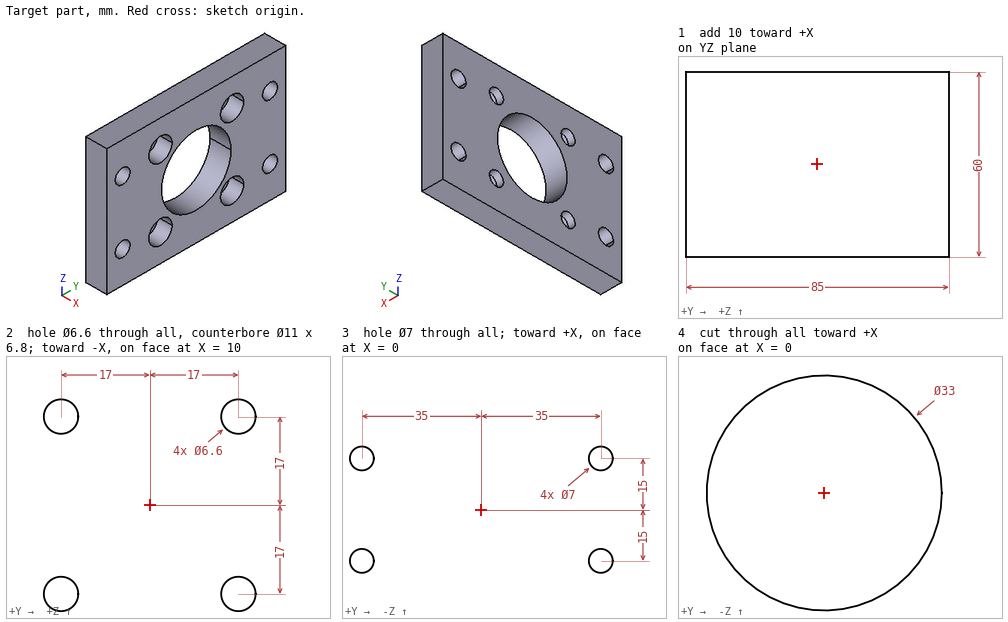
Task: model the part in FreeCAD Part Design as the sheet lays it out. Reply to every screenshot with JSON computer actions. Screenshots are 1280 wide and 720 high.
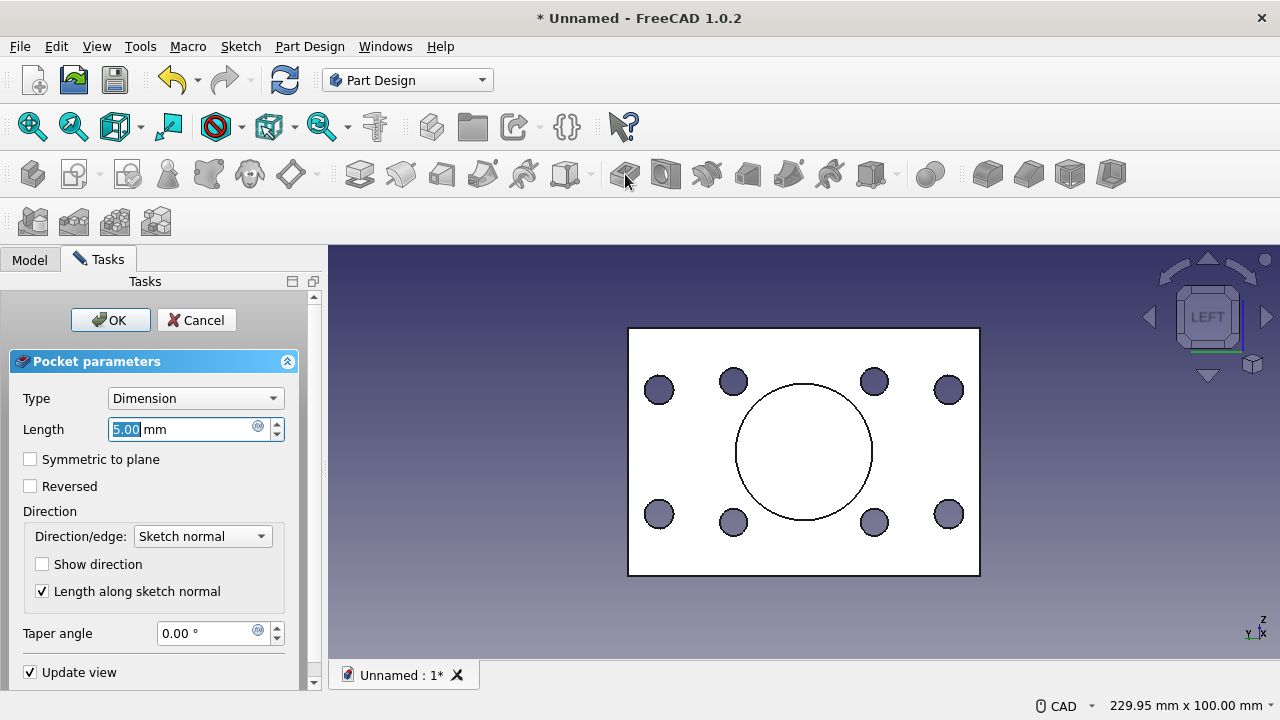
{"action": "left_click", "coordinate": [196, 398]}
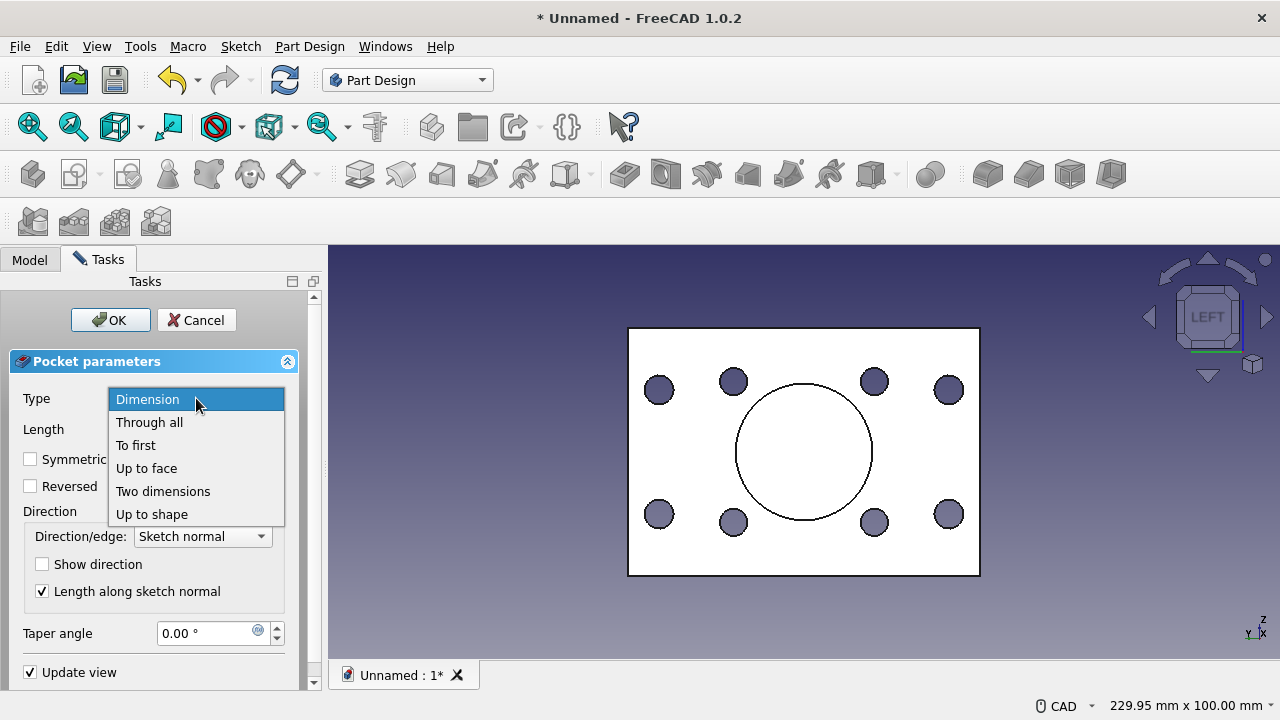
{"action": "left_click", "coordinate": [194, 422]}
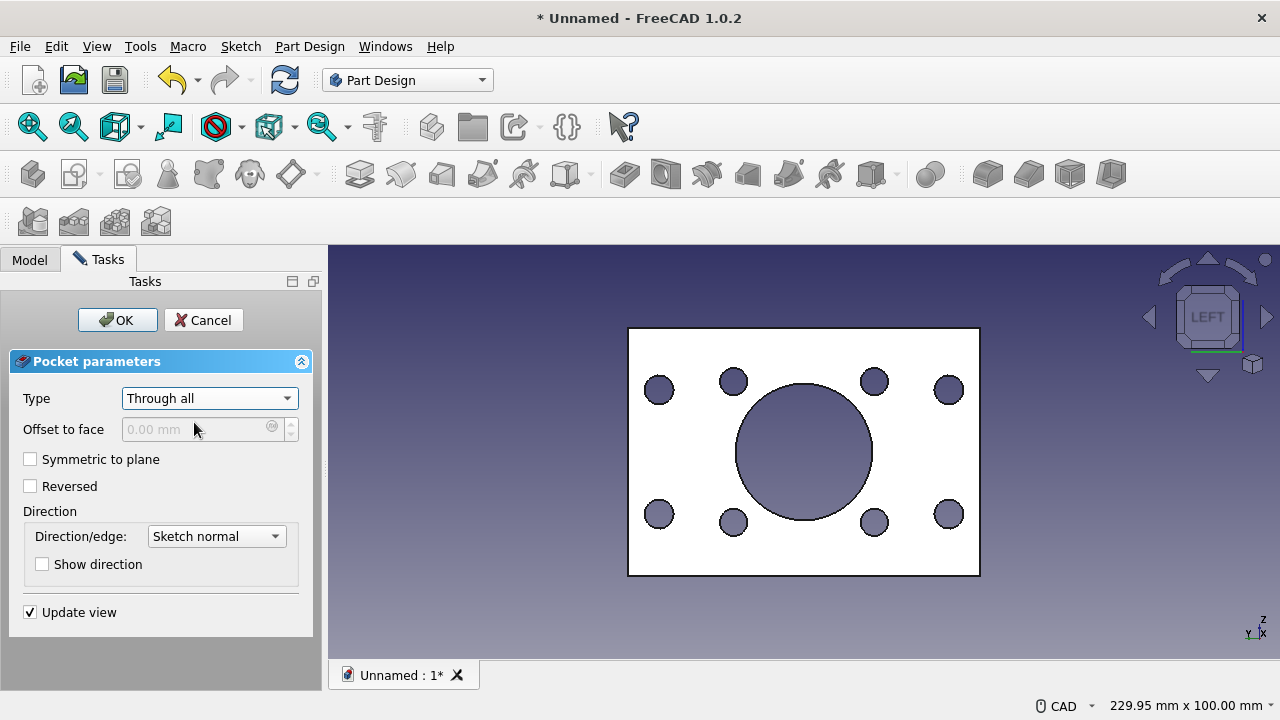
{"action": "left_click", "coordinate": [118, 320]}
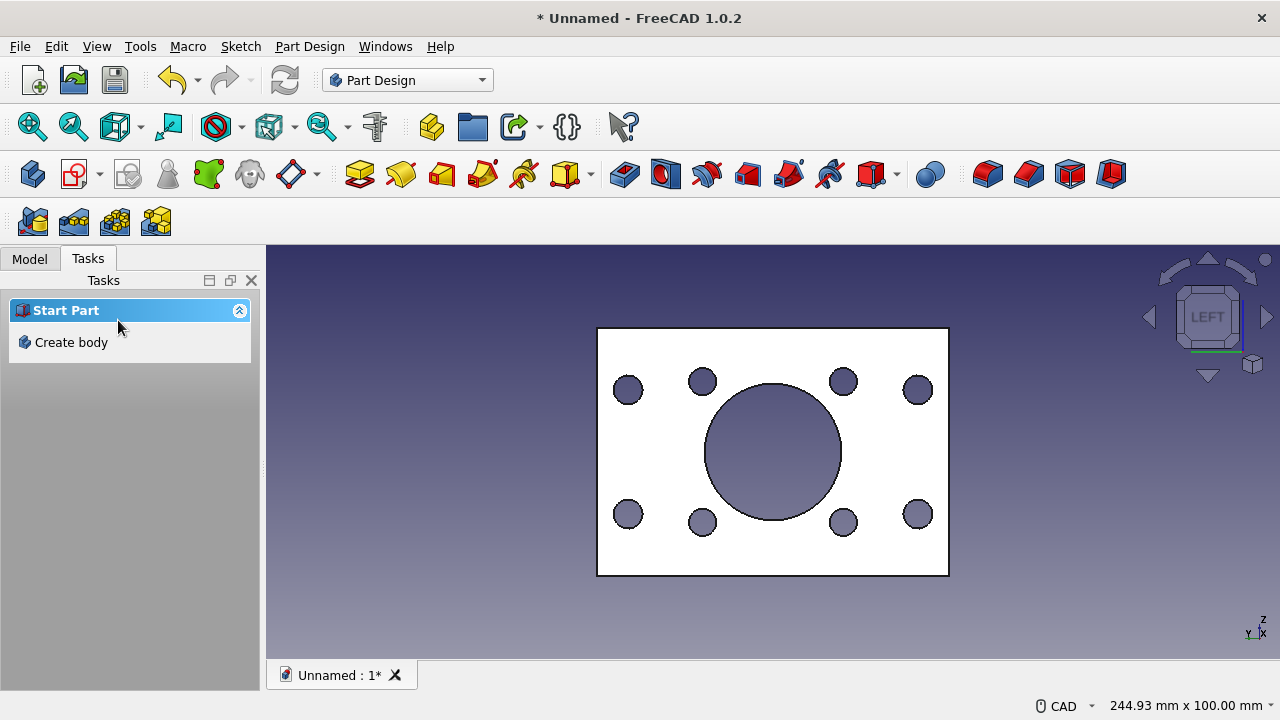
{"action": "key", "text": "0"}